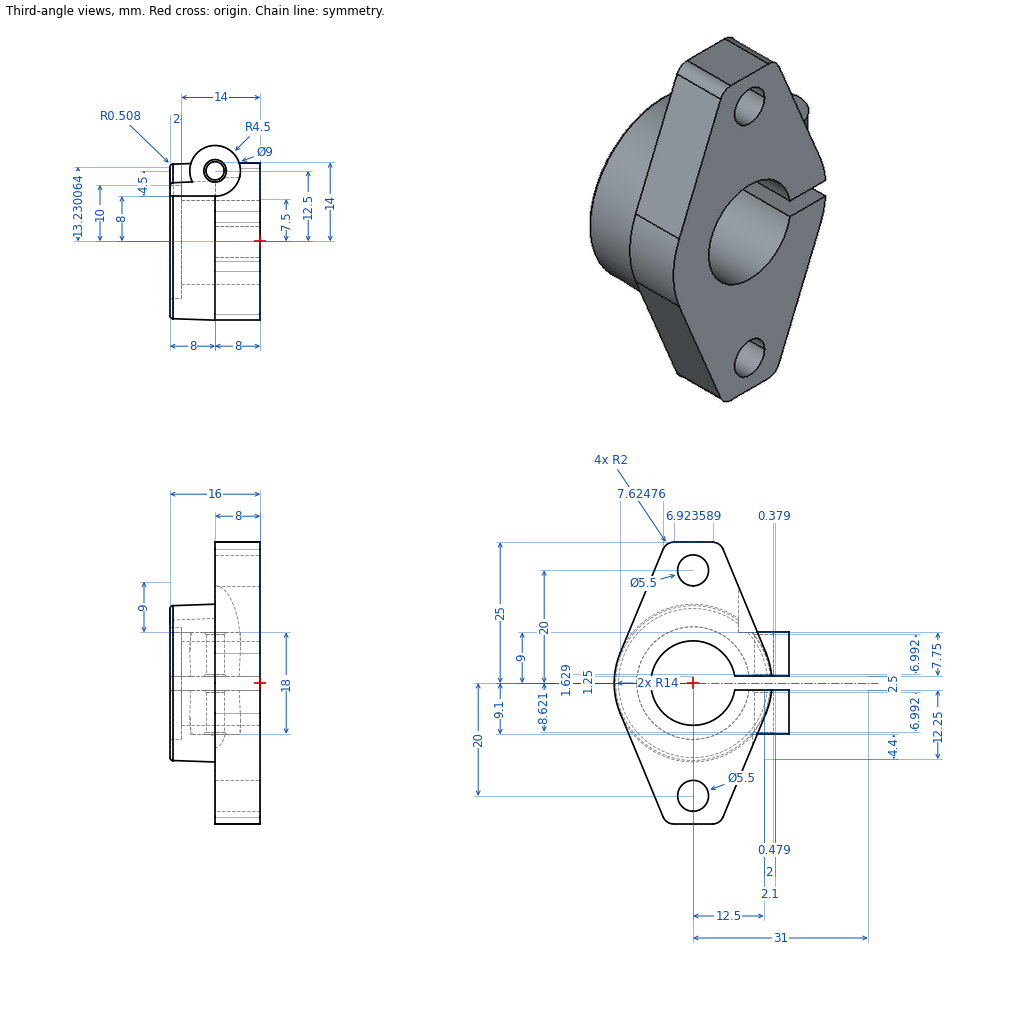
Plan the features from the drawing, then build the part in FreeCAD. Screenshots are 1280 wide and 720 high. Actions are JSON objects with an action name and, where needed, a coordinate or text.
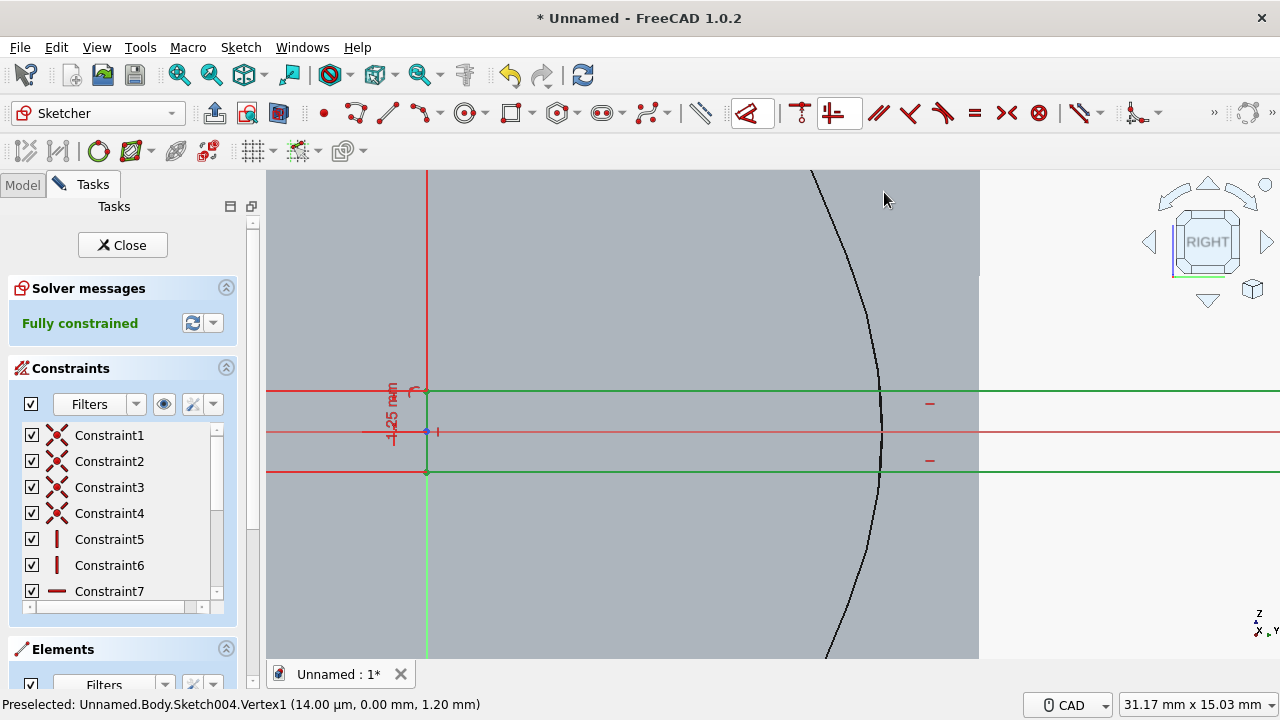
{"action": "left_click", "coordinate": [123, 245]}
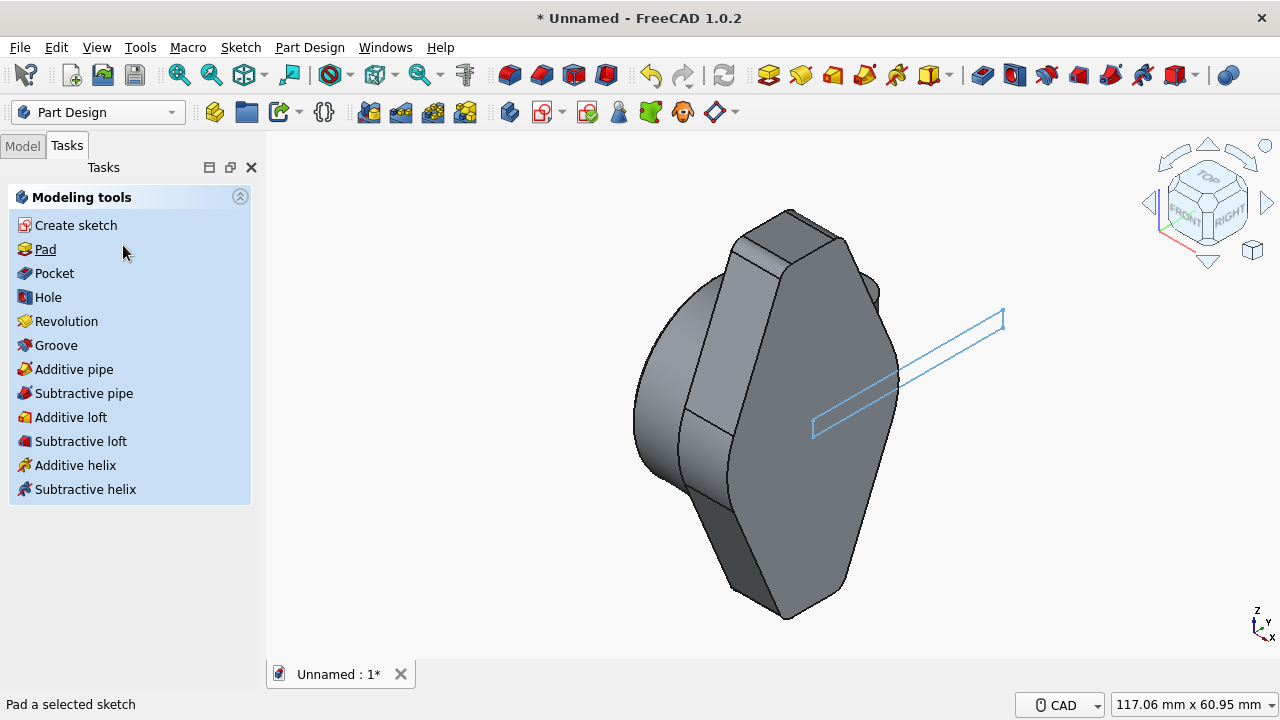
{"action": "left_click", "coordinate": [984, 76]}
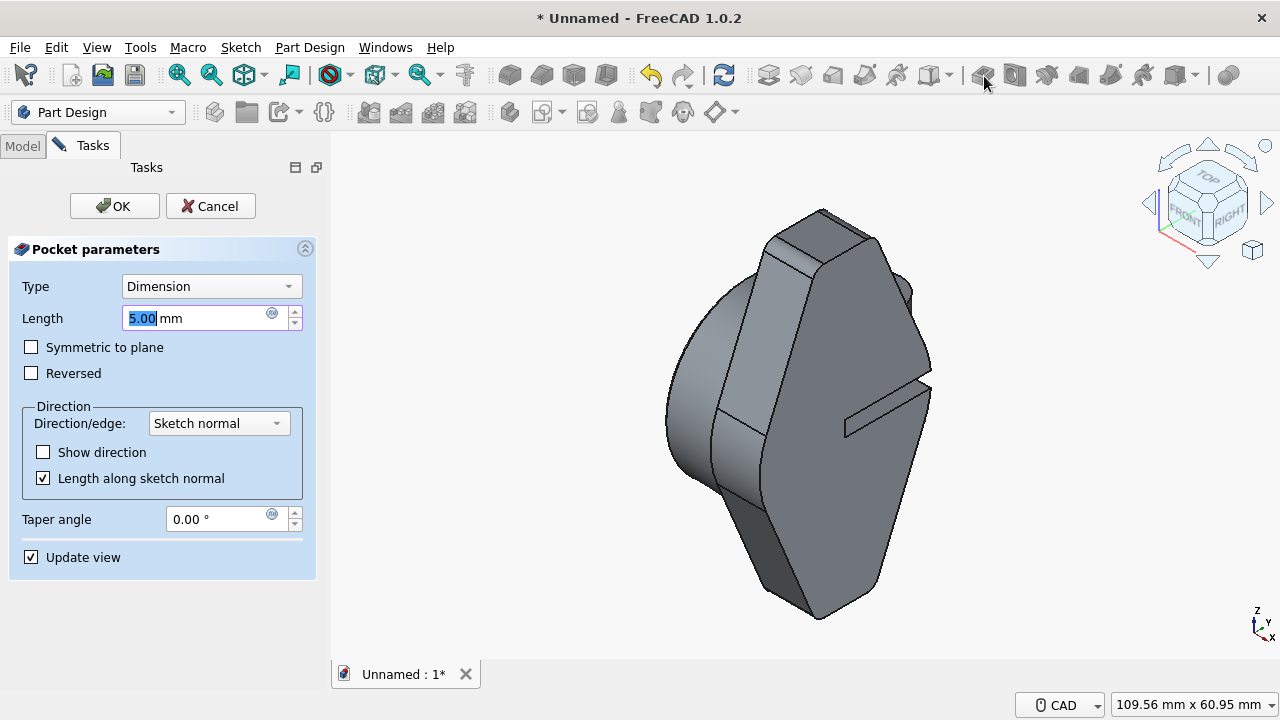
{"action": "type", "text": "16"}
{"action": "key", "text": "Tab"}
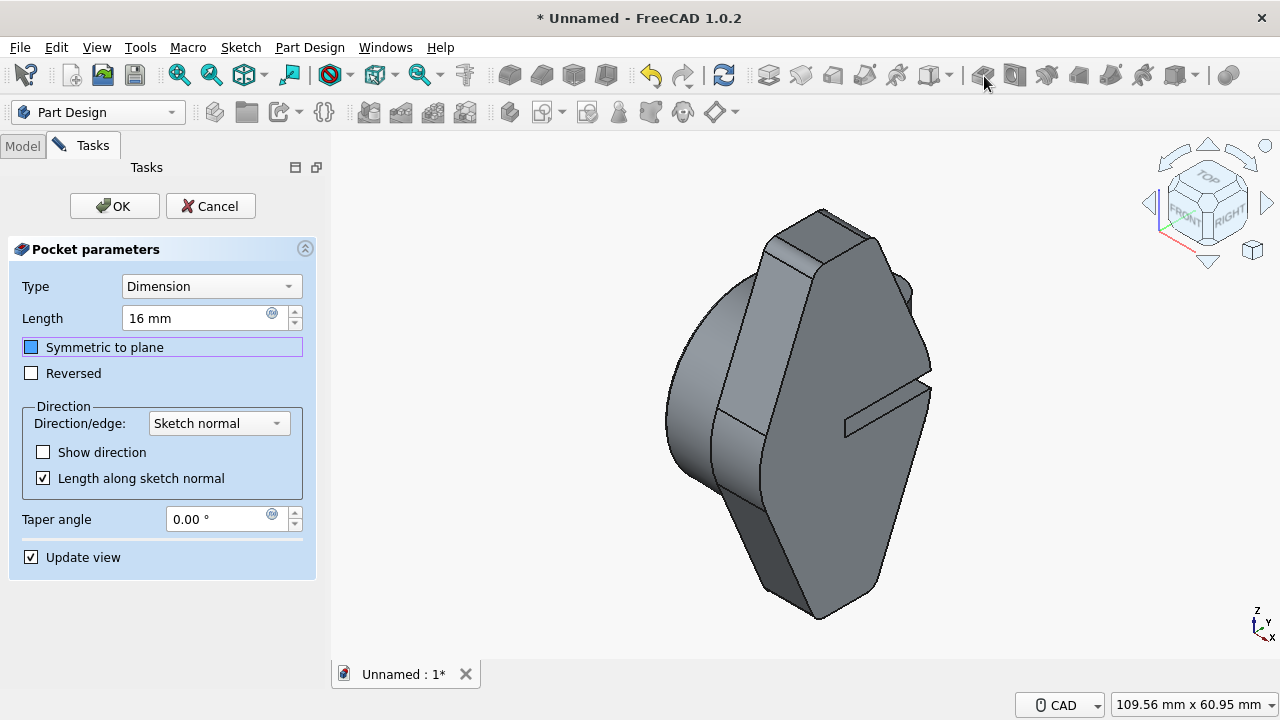
{"action": "left_click", "coordinate": [115, 206]}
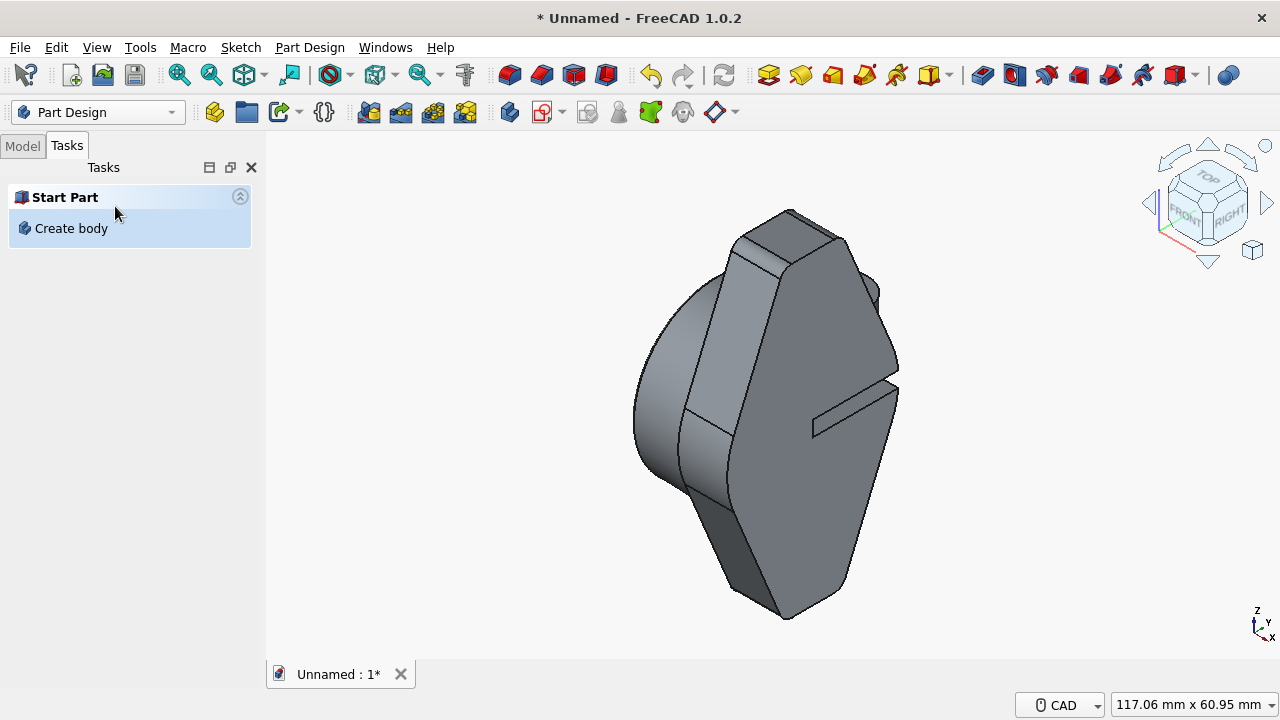
{"action": "left_click", "coordinate": [542, 112]}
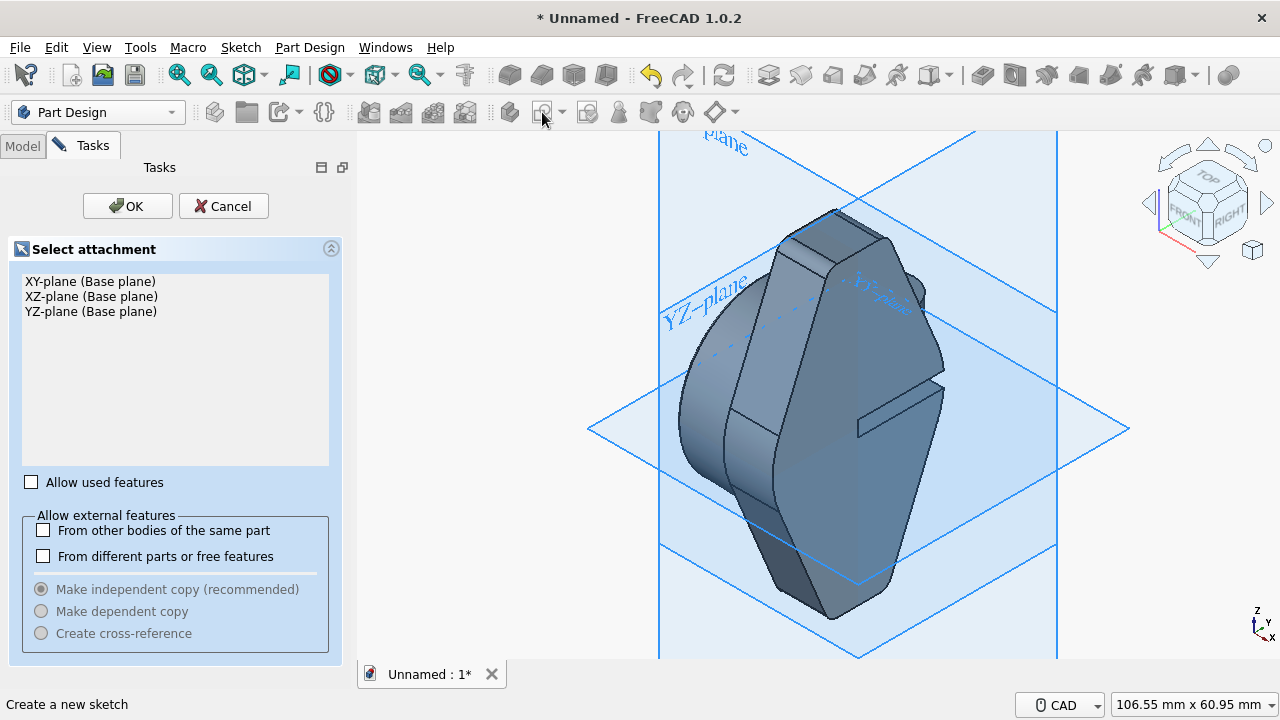
{"action": "left_click", "coordinate": [82, 282]}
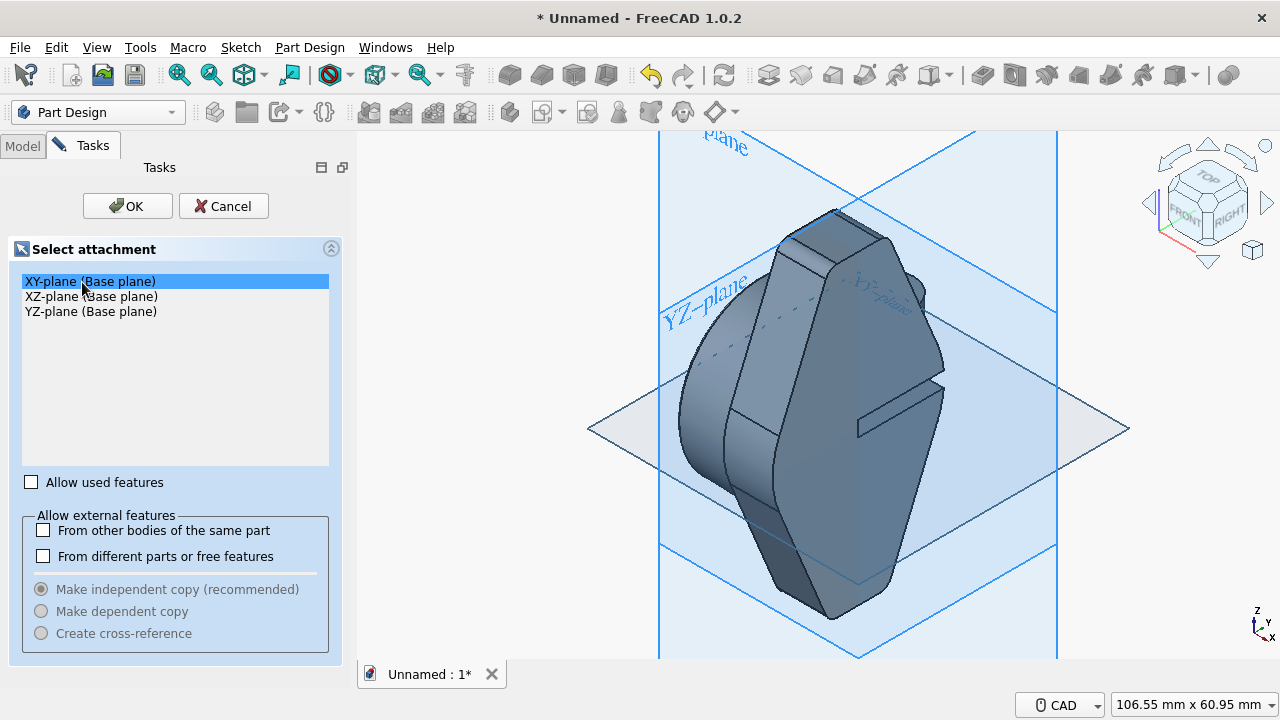
{"action": "left_click", "coordinate": [128, 206]}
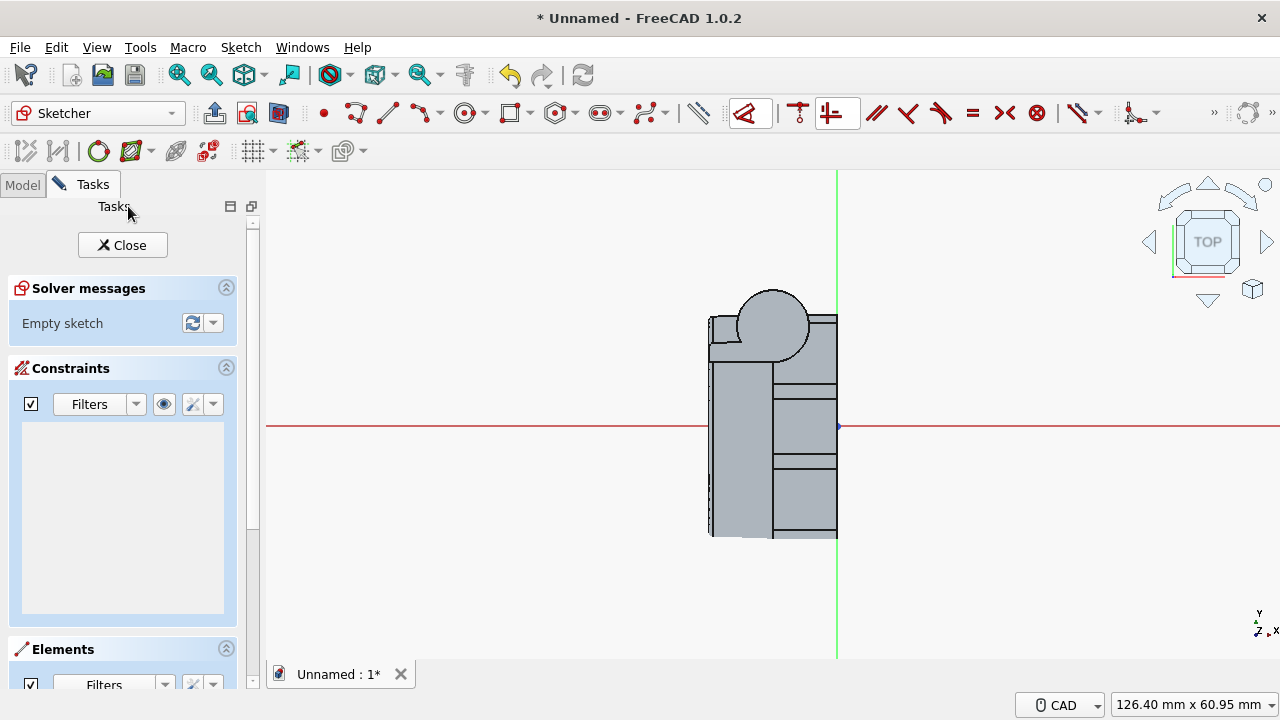
{"action": "left_click", "coordinate": [280, 114]}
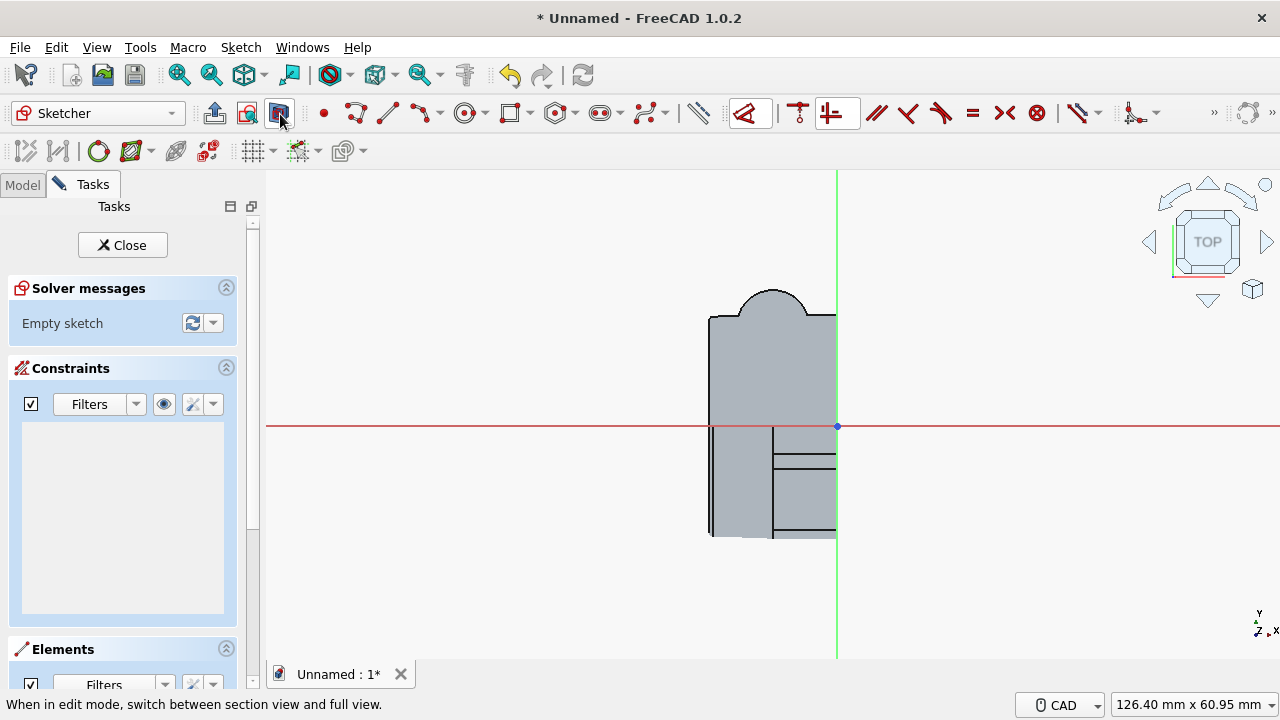
{"action": "scroll", "coordinate": [795, 377], "scroll_direction": "up", "scroll_amount": 7}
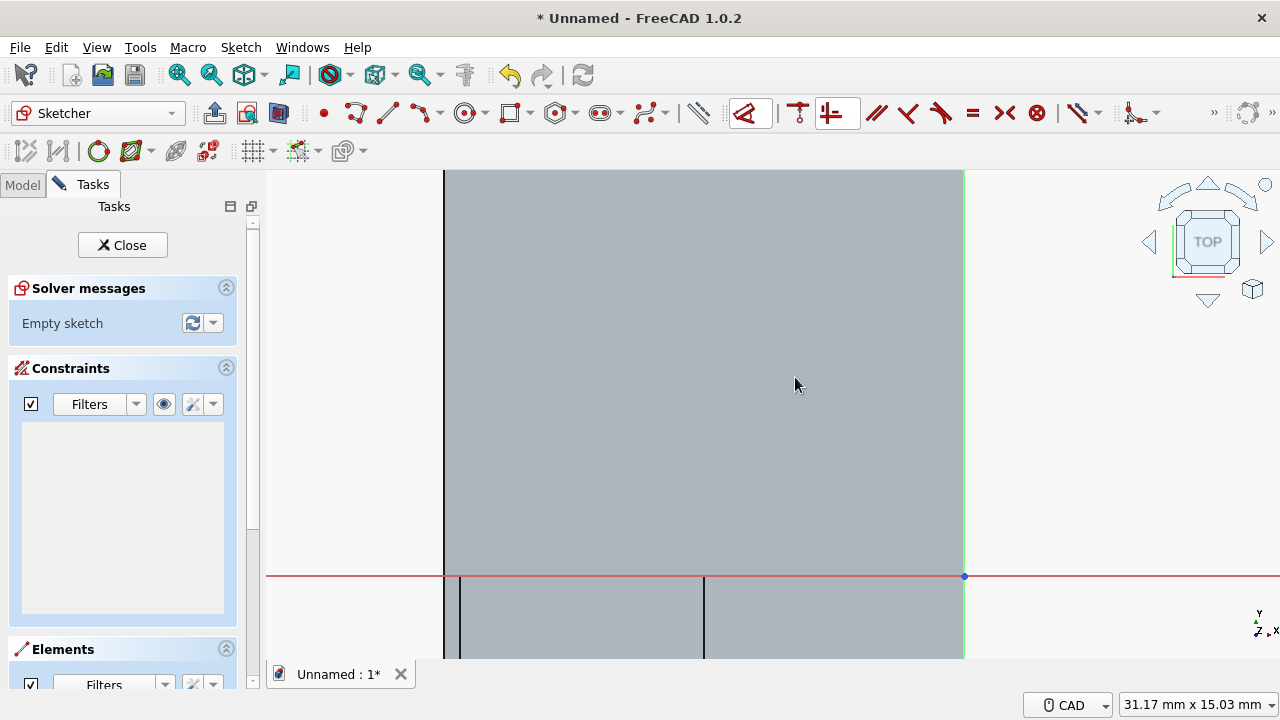
{"action": "key", "text": "g m"}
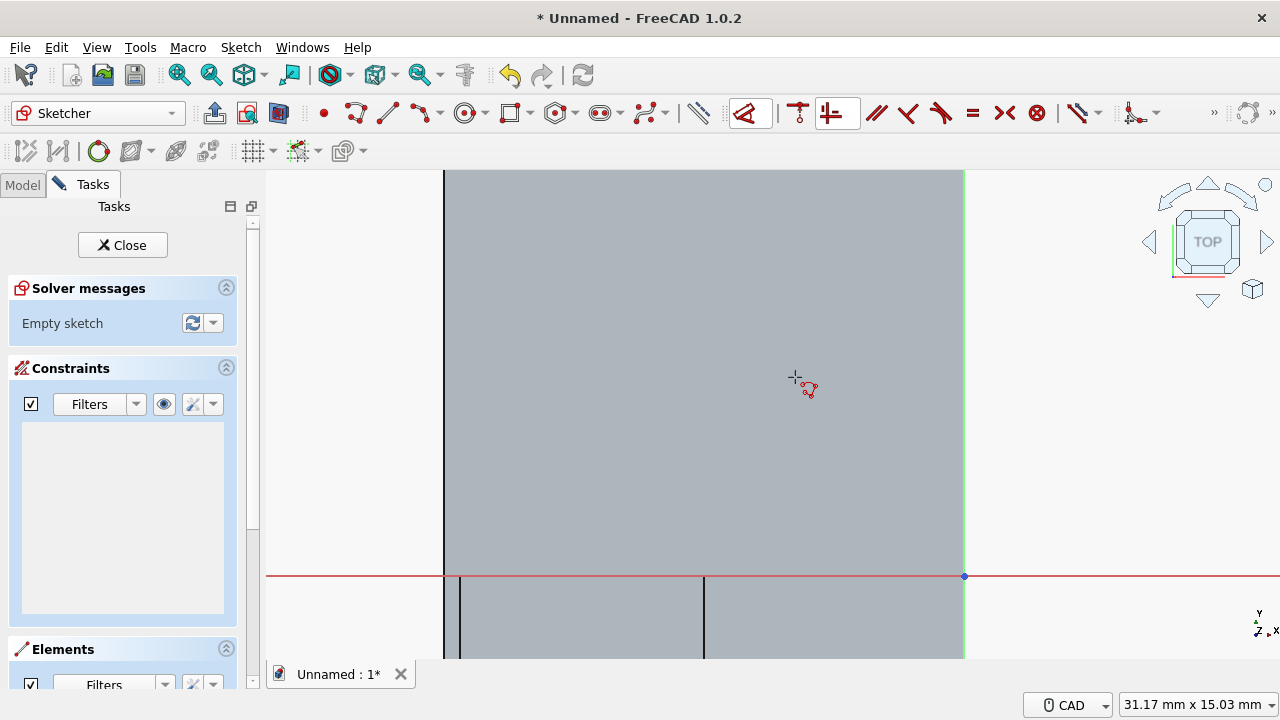
{"action": "left_click", "coordinate": [964, 576]}
{"action": "left_click", "coordinate": [955, 332]}
{"action": "left_click", "coordinate": [509, 332]}
{"action": "left_click", "coordinate": [509, 251]}
{"action": "left_click", "coordinate": [444, 251]}
{"action": "left_click", "coordinate": [444, 567]}
{"action": "left_click", "coordinate": [964, 576]}
{"action": "key", "text": "Escape"}
{"action": "key", "text": "Escape"}